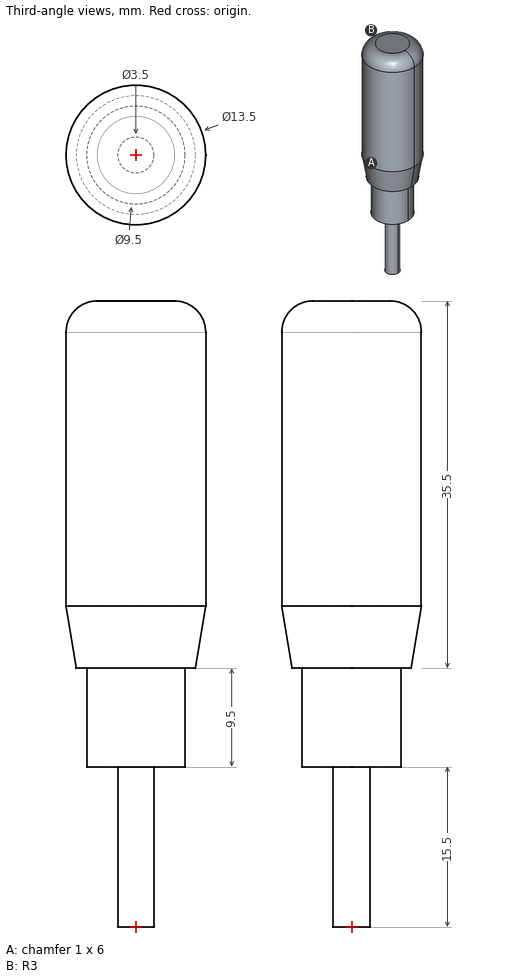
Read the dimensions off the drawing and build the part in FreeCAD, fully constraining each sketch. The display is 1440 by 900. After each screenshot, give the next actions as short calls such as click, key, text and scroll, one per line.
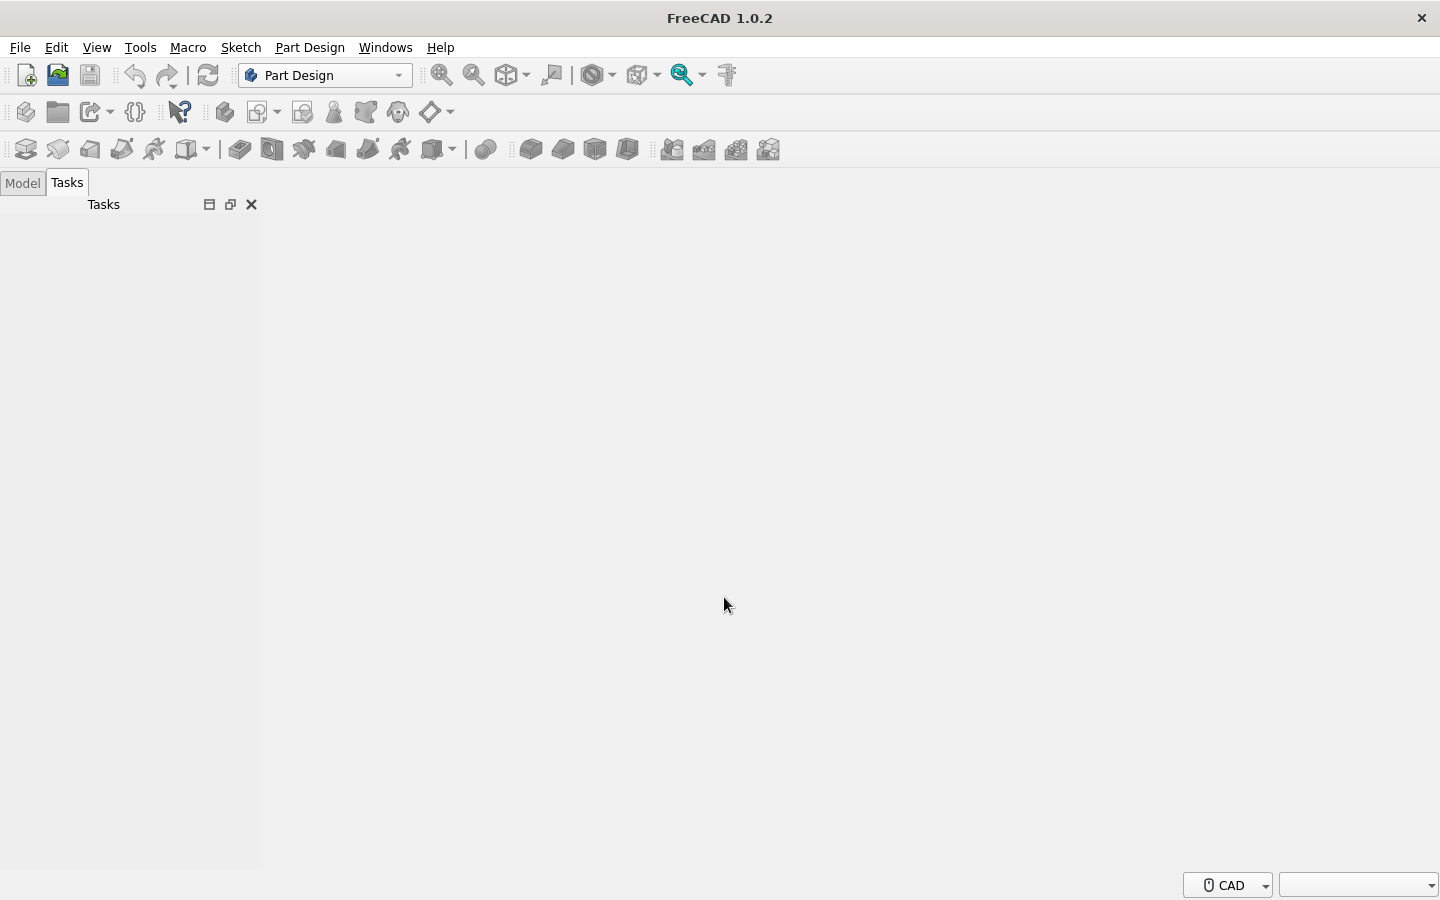
click(26, 76)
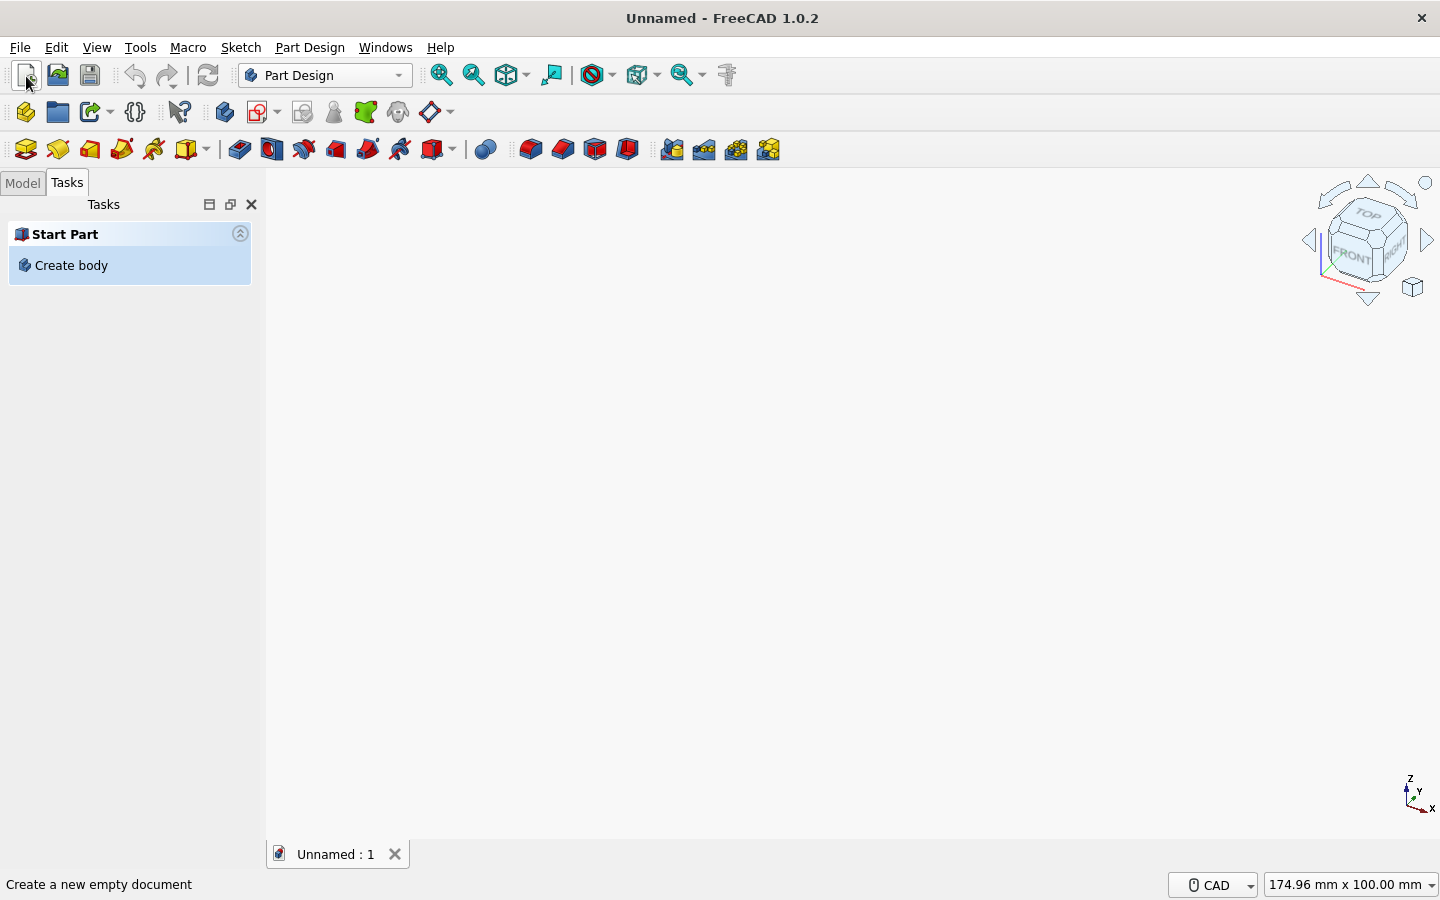
click(258, 112)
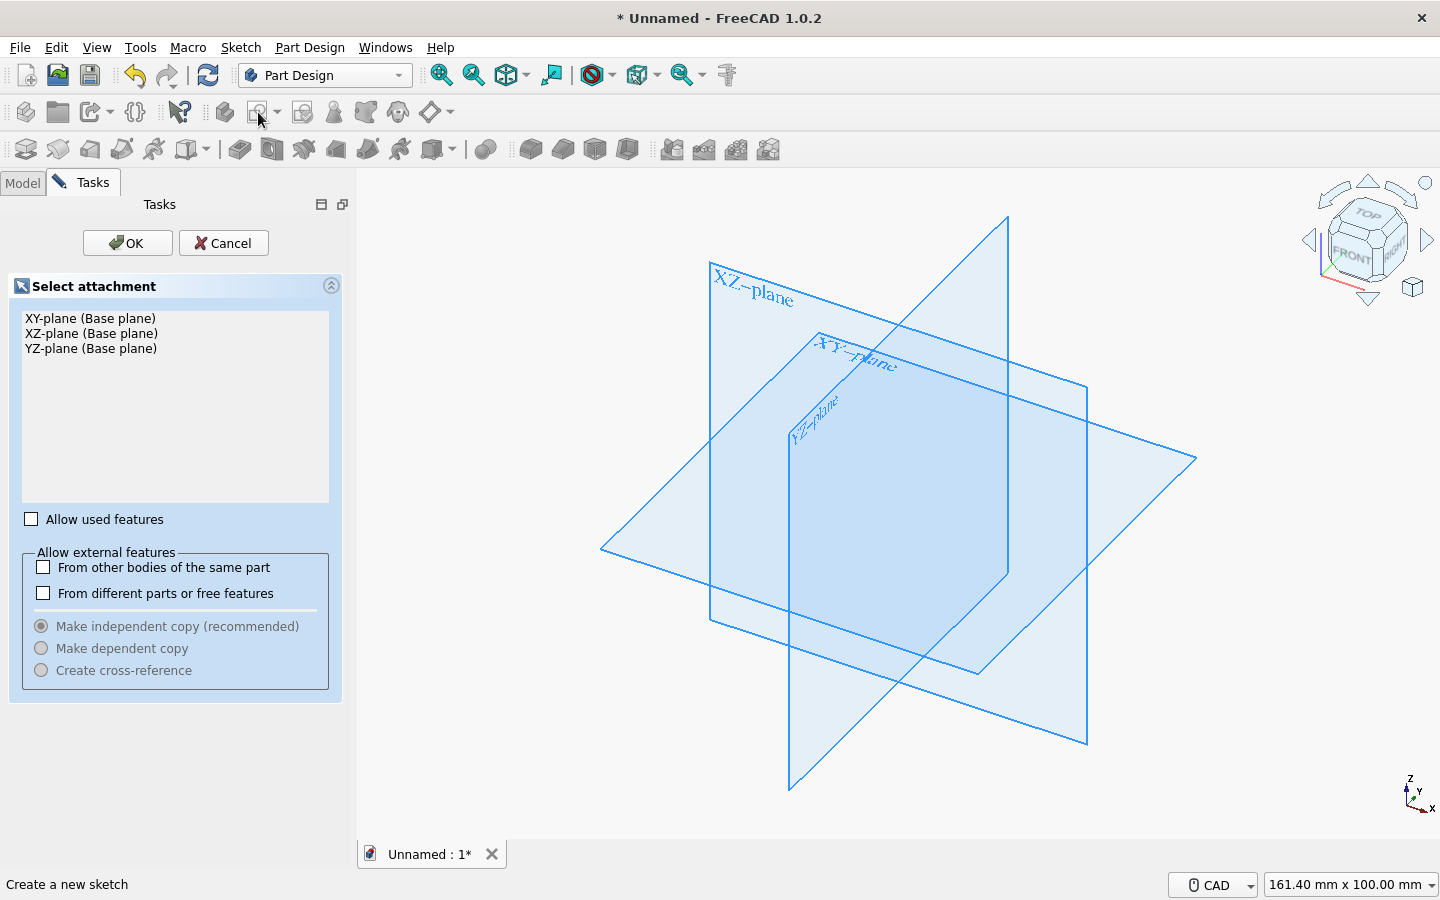
click(82, 318)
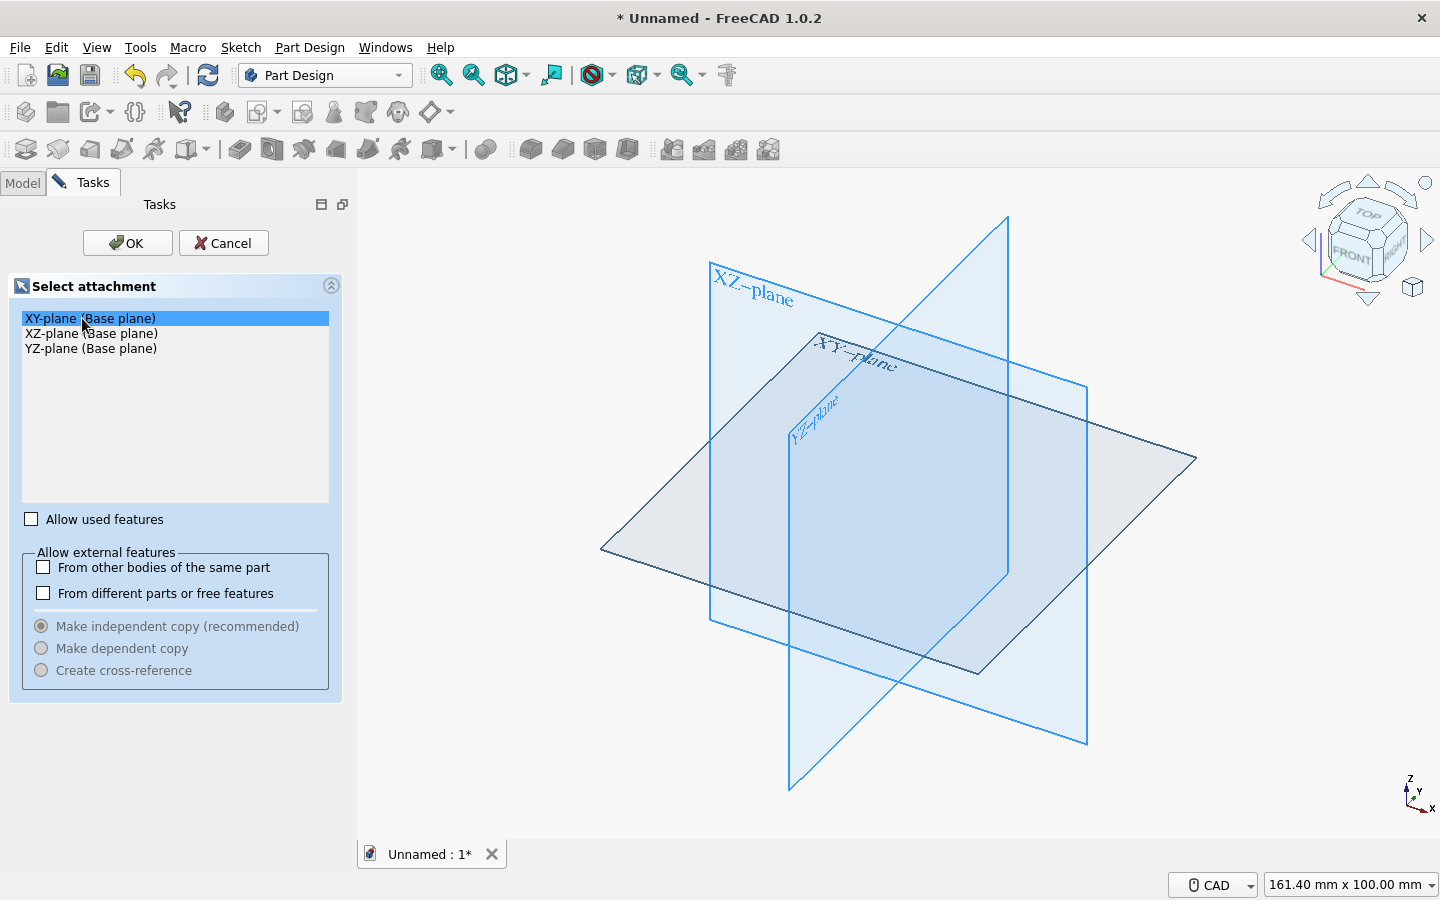
click(128, 243)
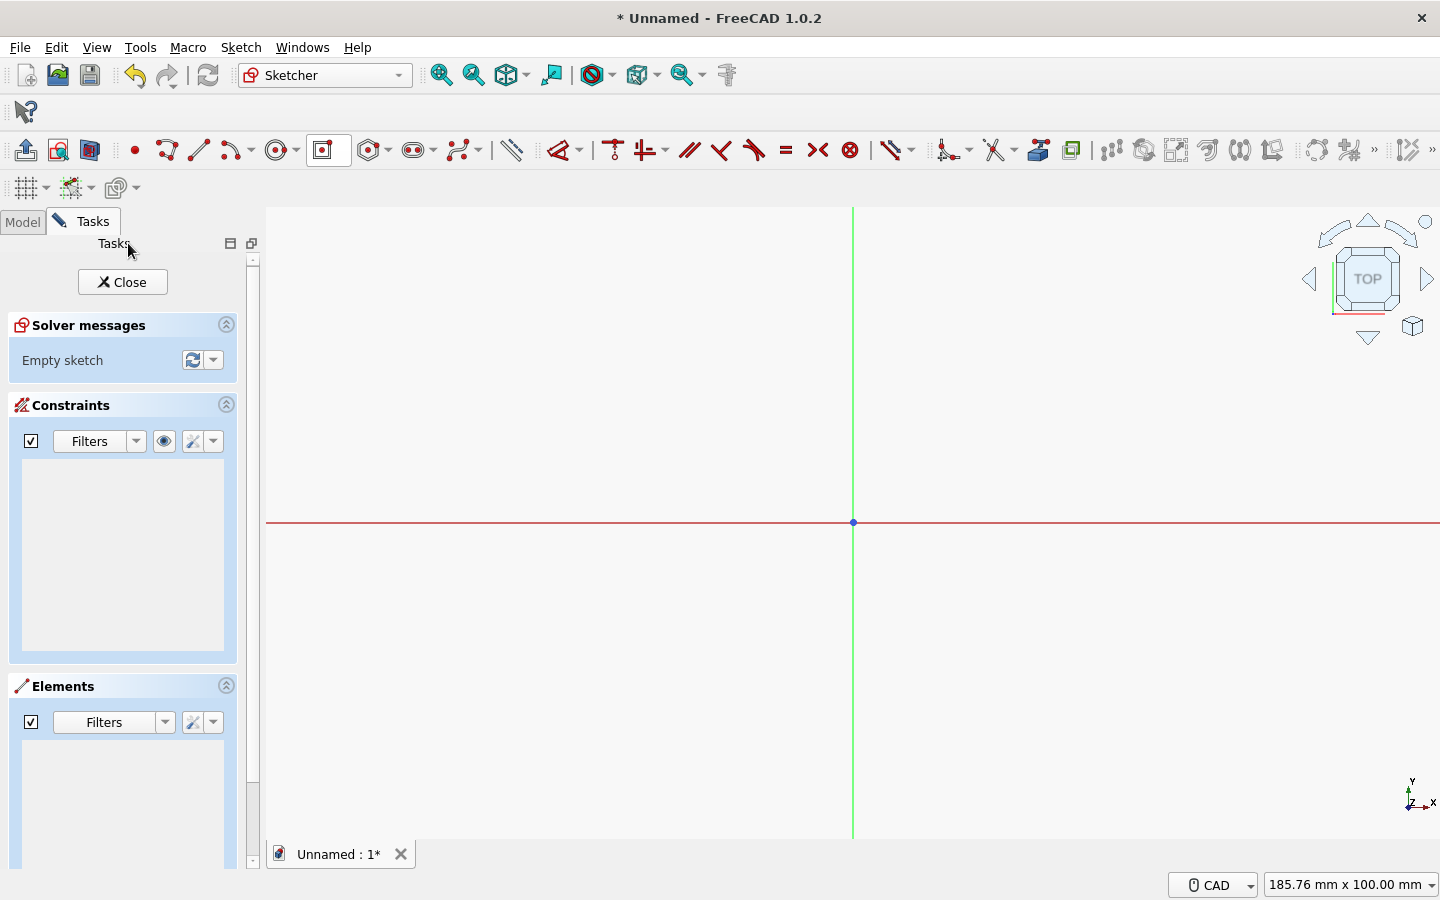
scroll(857, 523, up, 15)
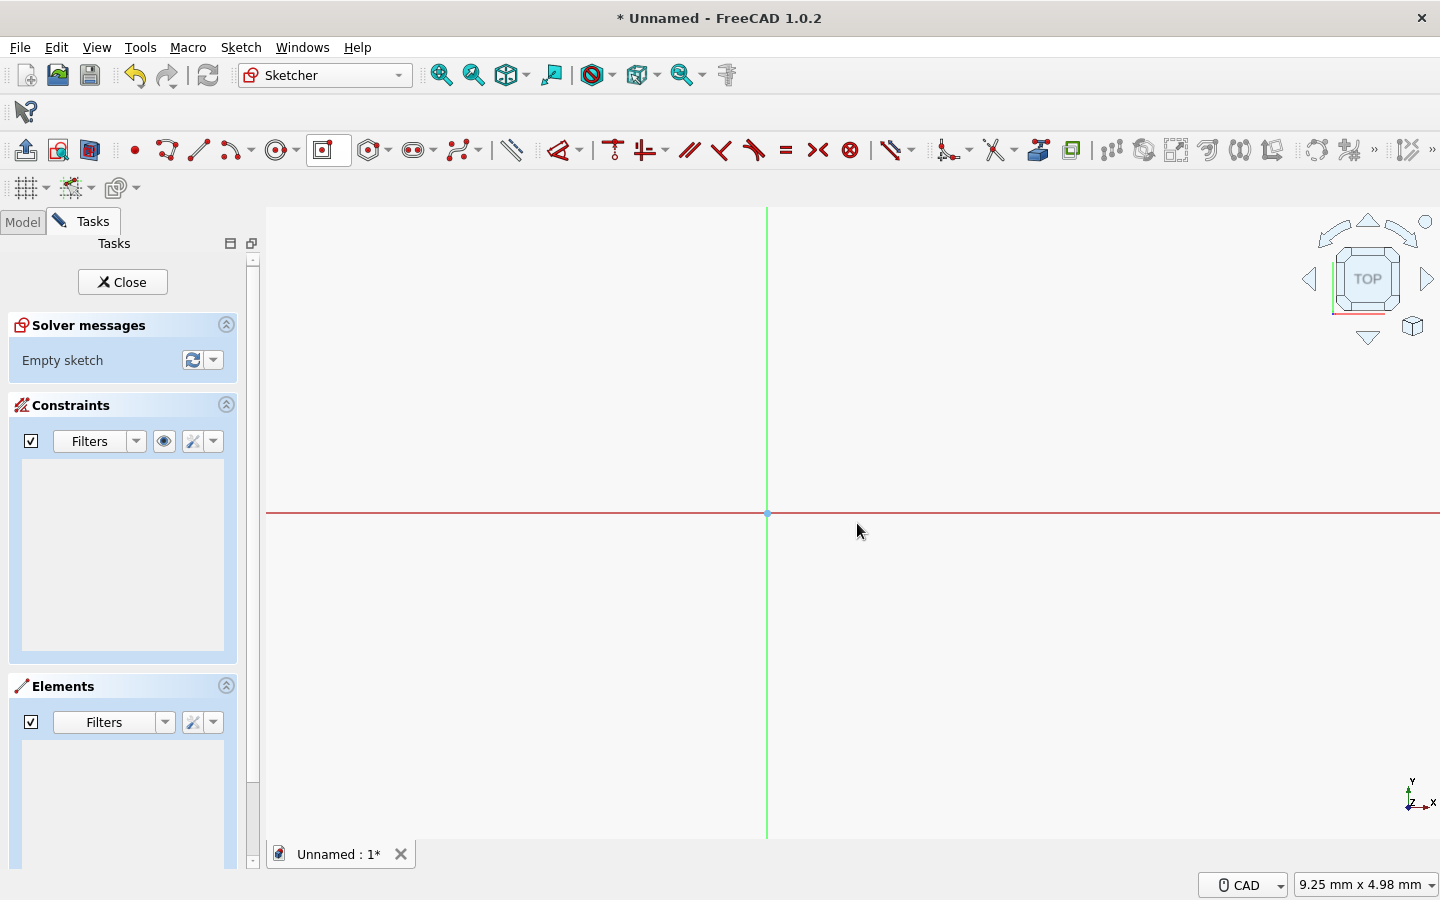
click(276, 150)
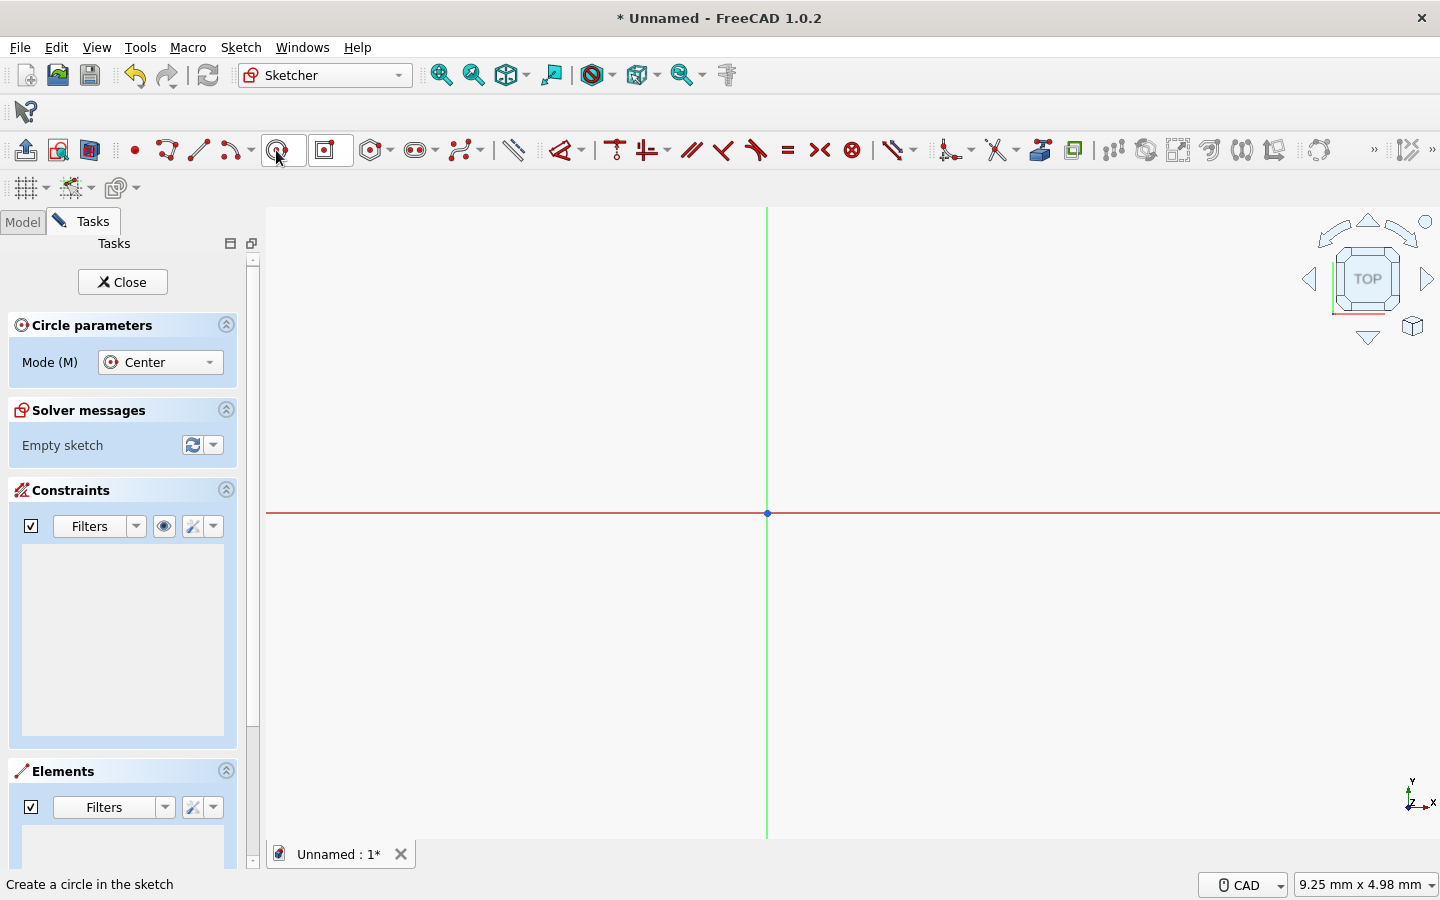
click(767, 513)
click(924, 356)
key(Escape)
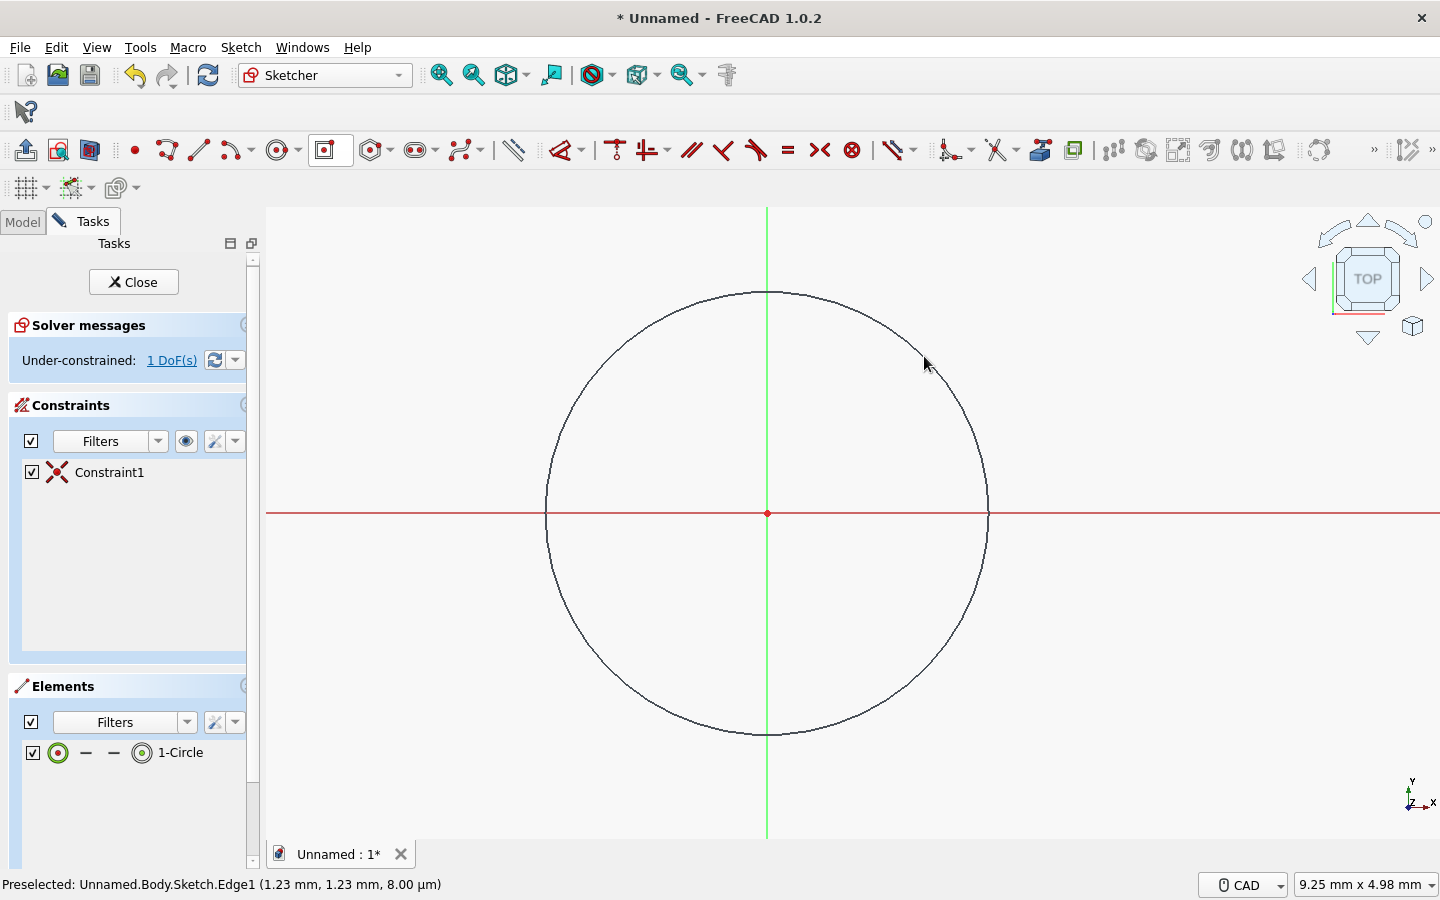
click(560, 150)